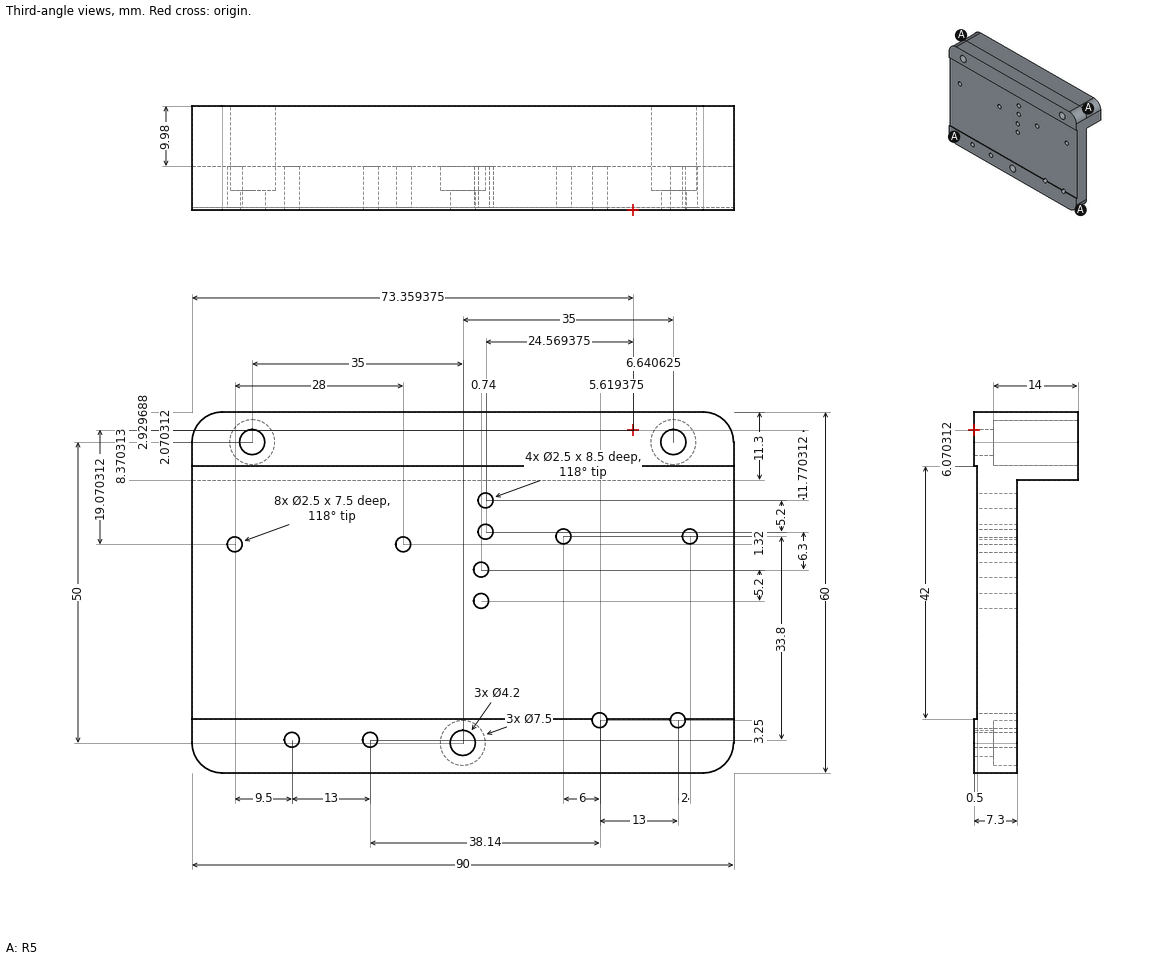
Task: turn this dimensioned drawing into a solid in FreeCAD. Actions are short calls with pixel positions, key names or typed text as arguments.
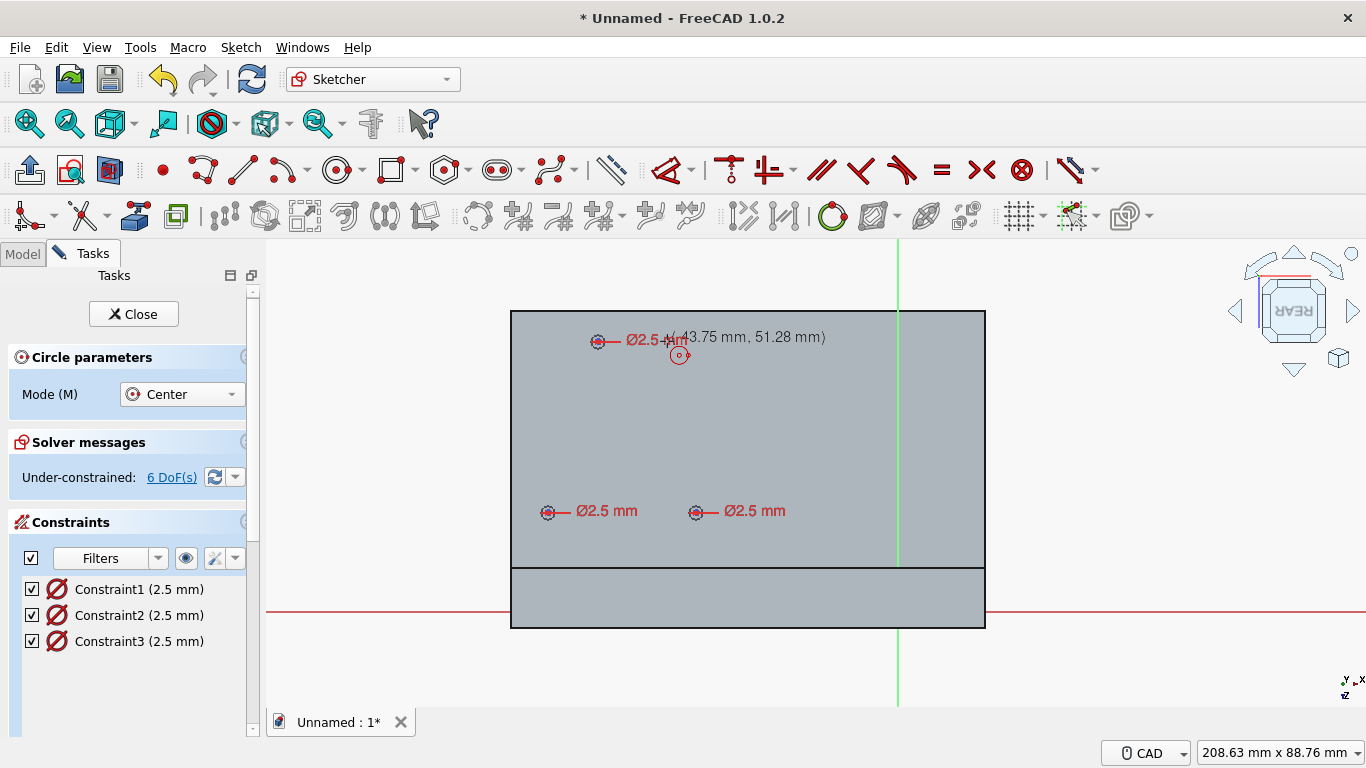
click(667, 341)
move(672, 336)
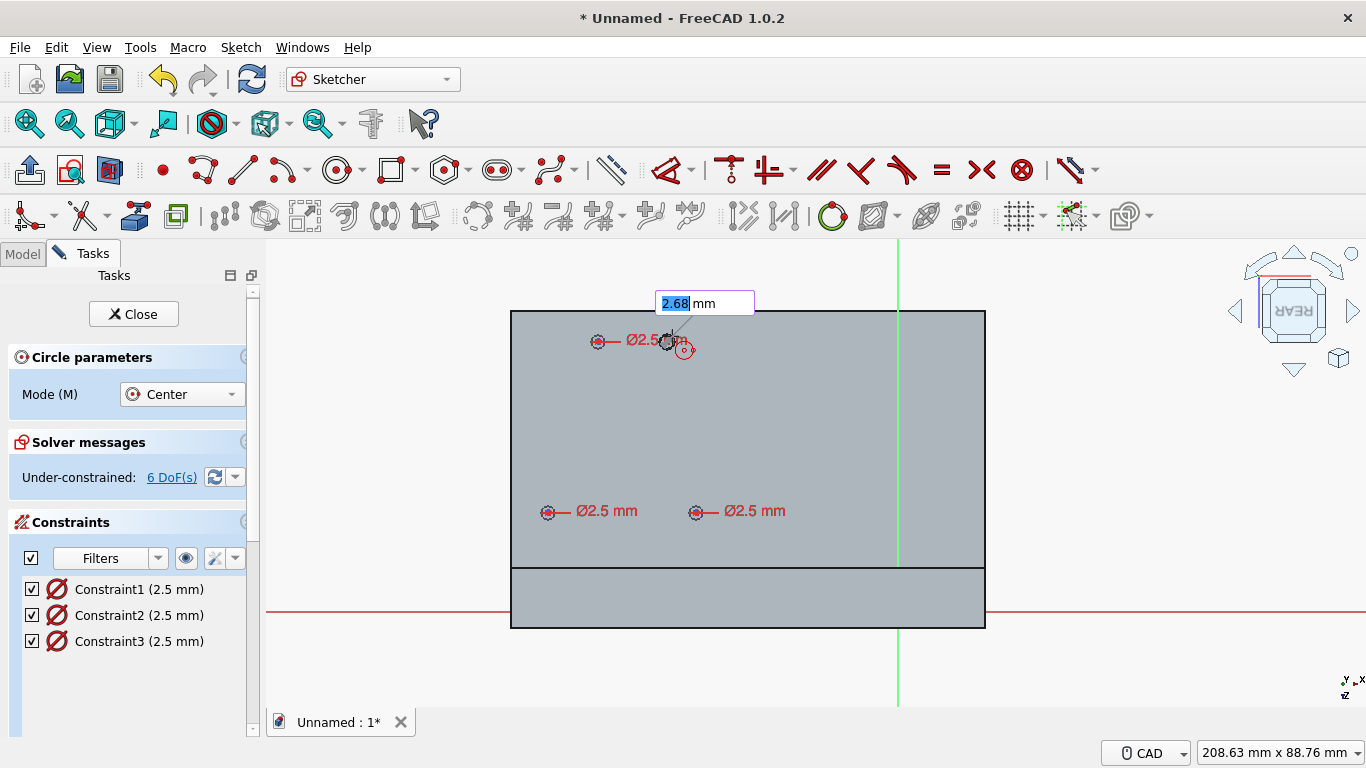
text(2.5)
key(Return)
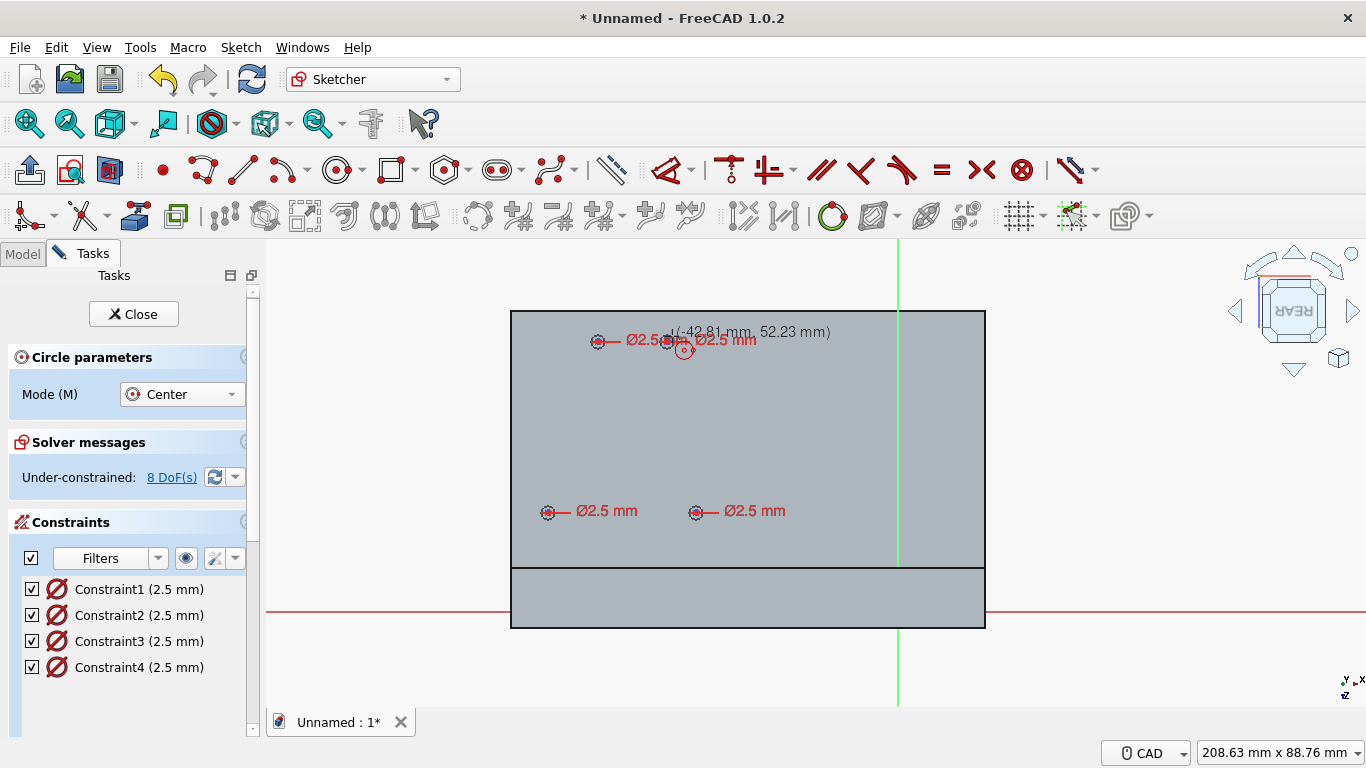
scroll(868, 358, up, 7)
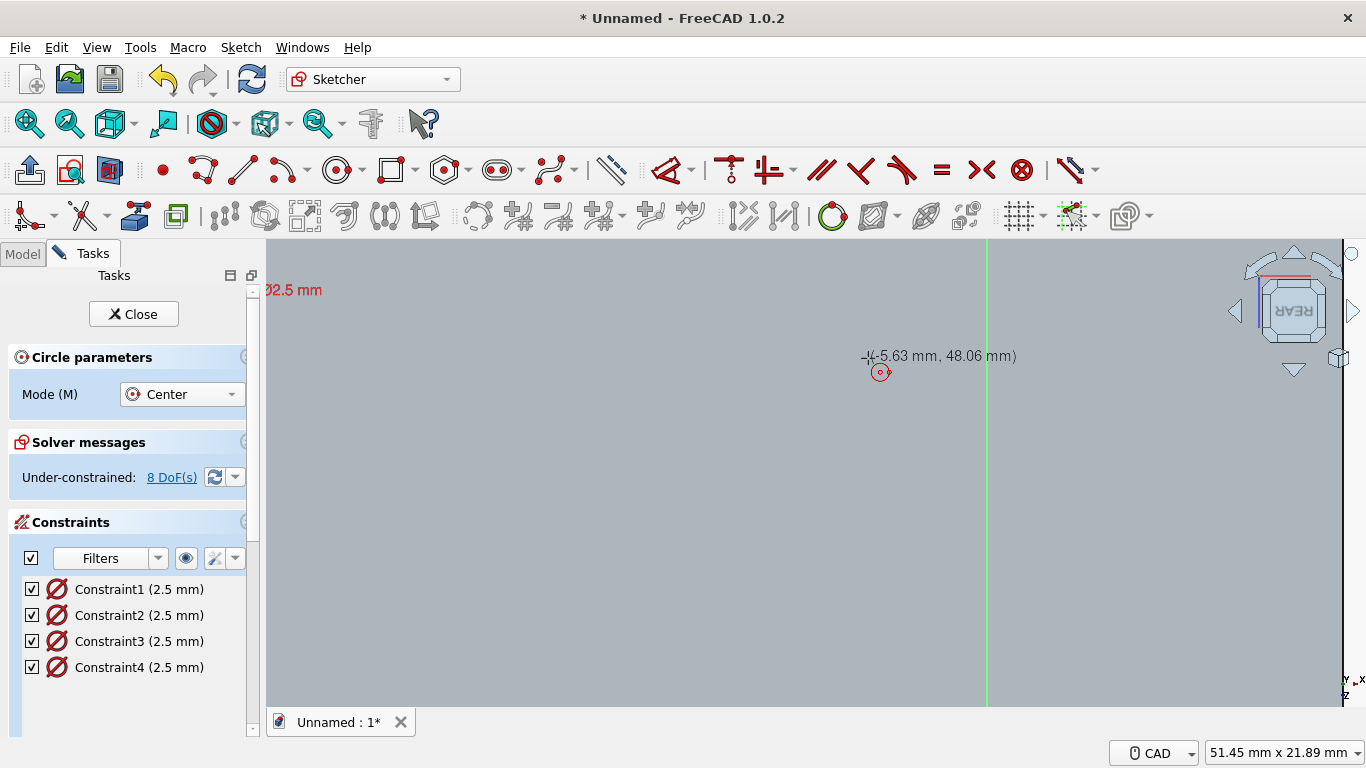
scroll(868, 358, down, 7)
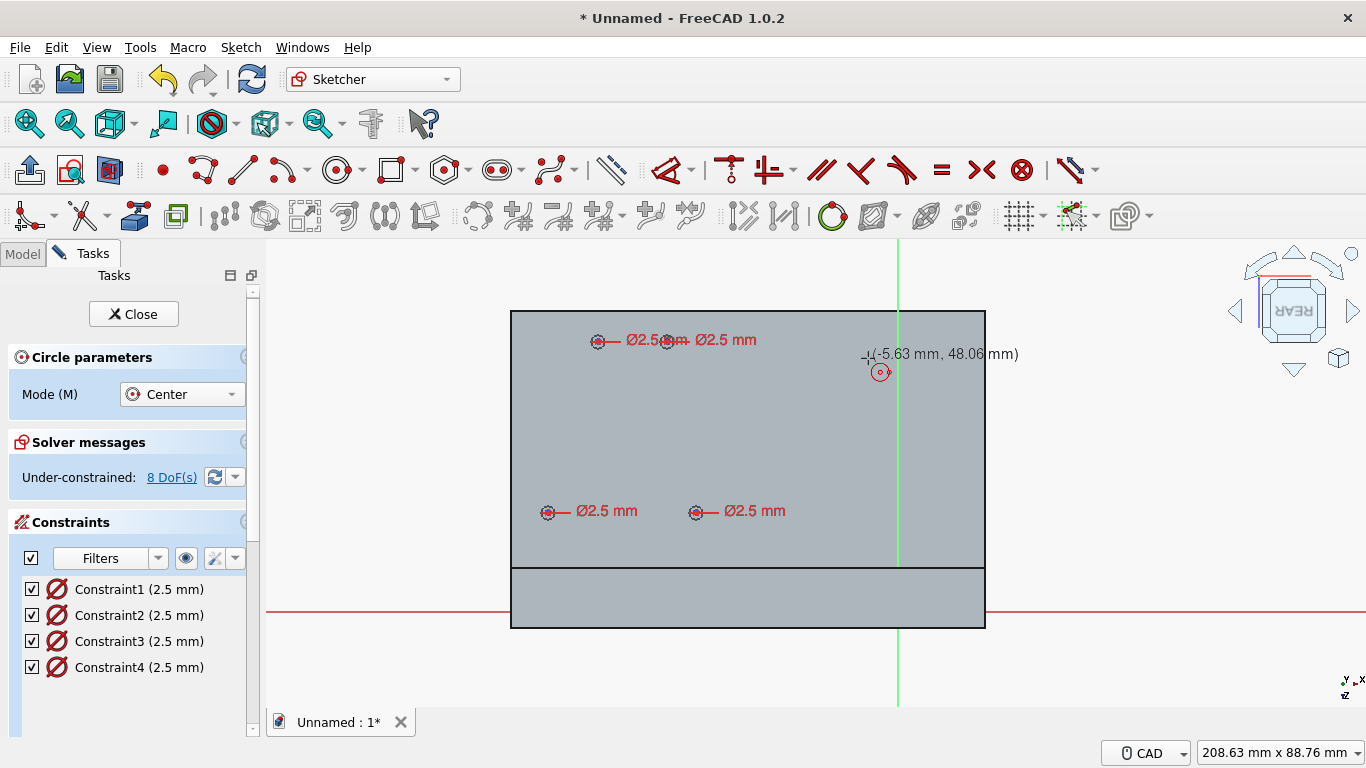
click(868, 358)
move(873, 353)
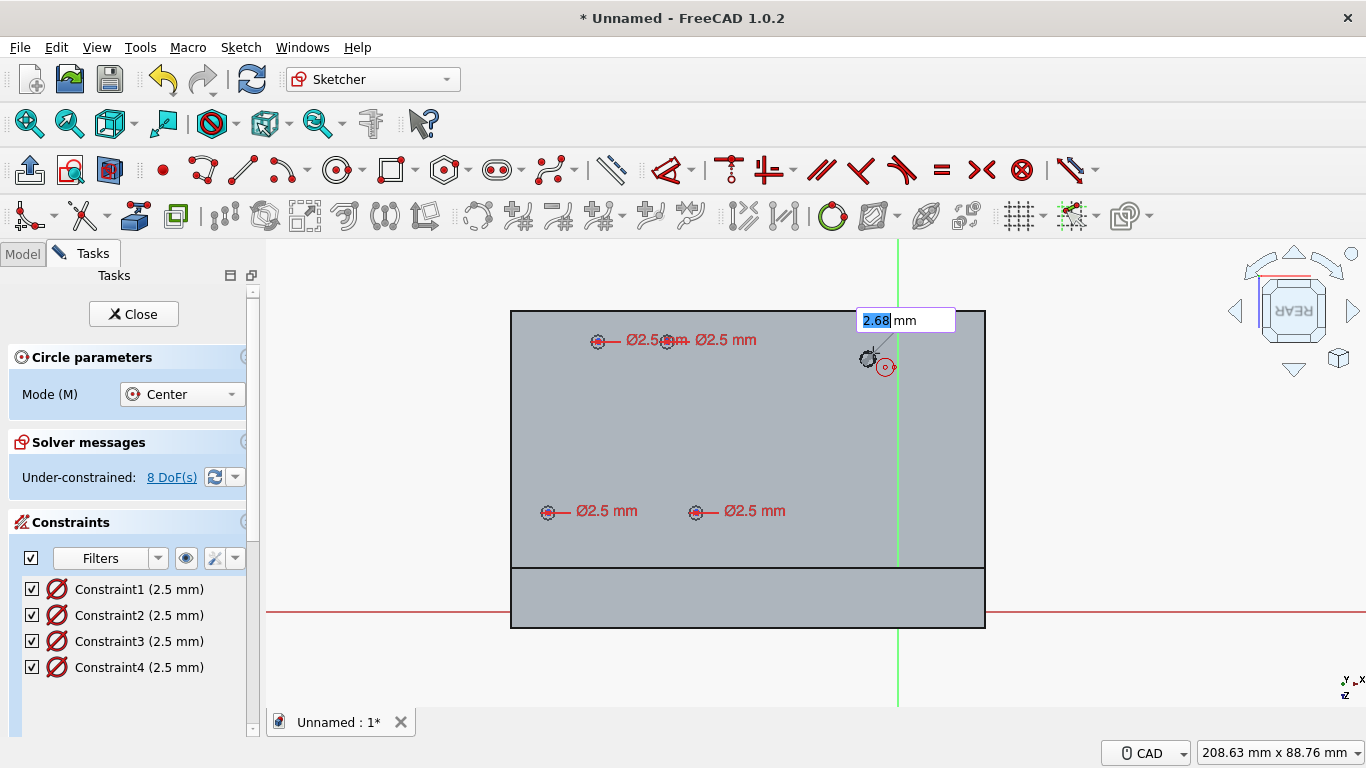
text(2.5)
key(Return)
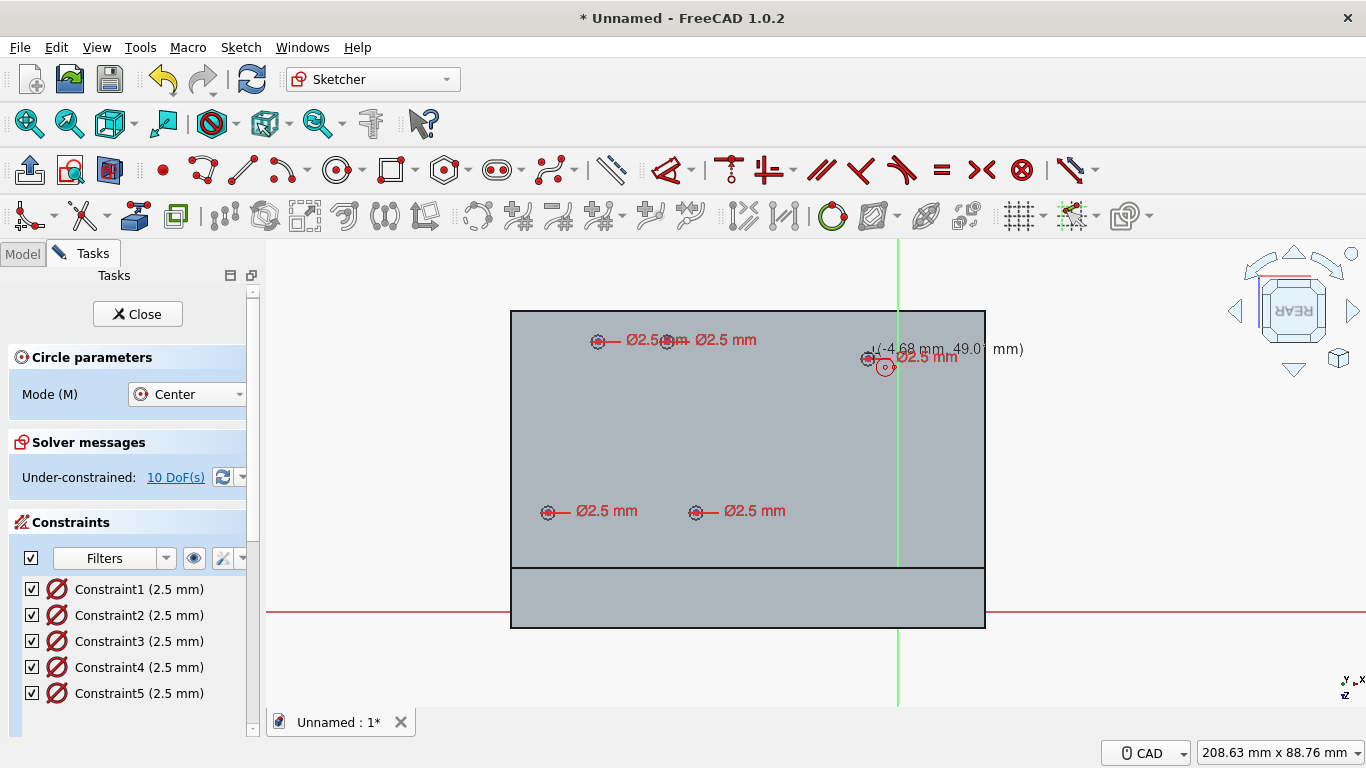
scroll(937, 358, up, 7)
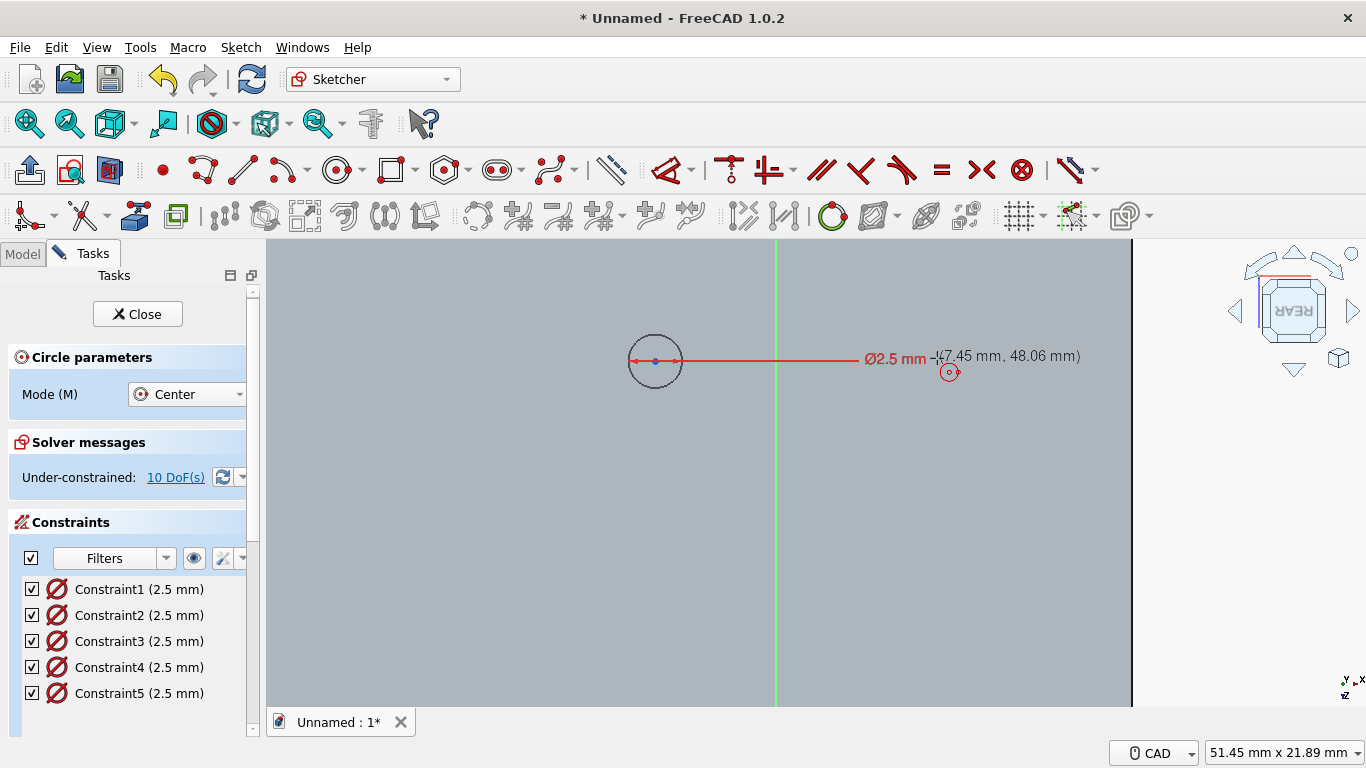
scroll(937, 358, down, 7)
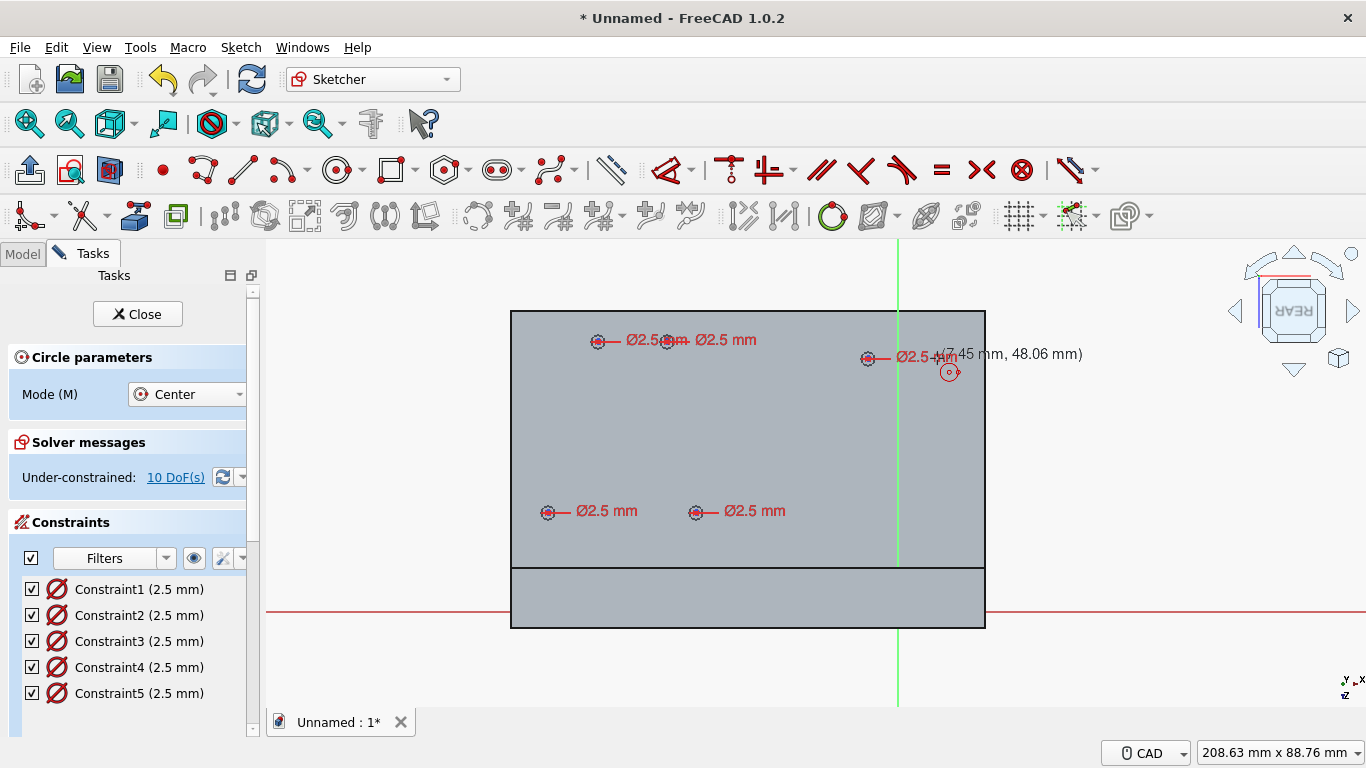
click(937, 358)
move(941, 353)